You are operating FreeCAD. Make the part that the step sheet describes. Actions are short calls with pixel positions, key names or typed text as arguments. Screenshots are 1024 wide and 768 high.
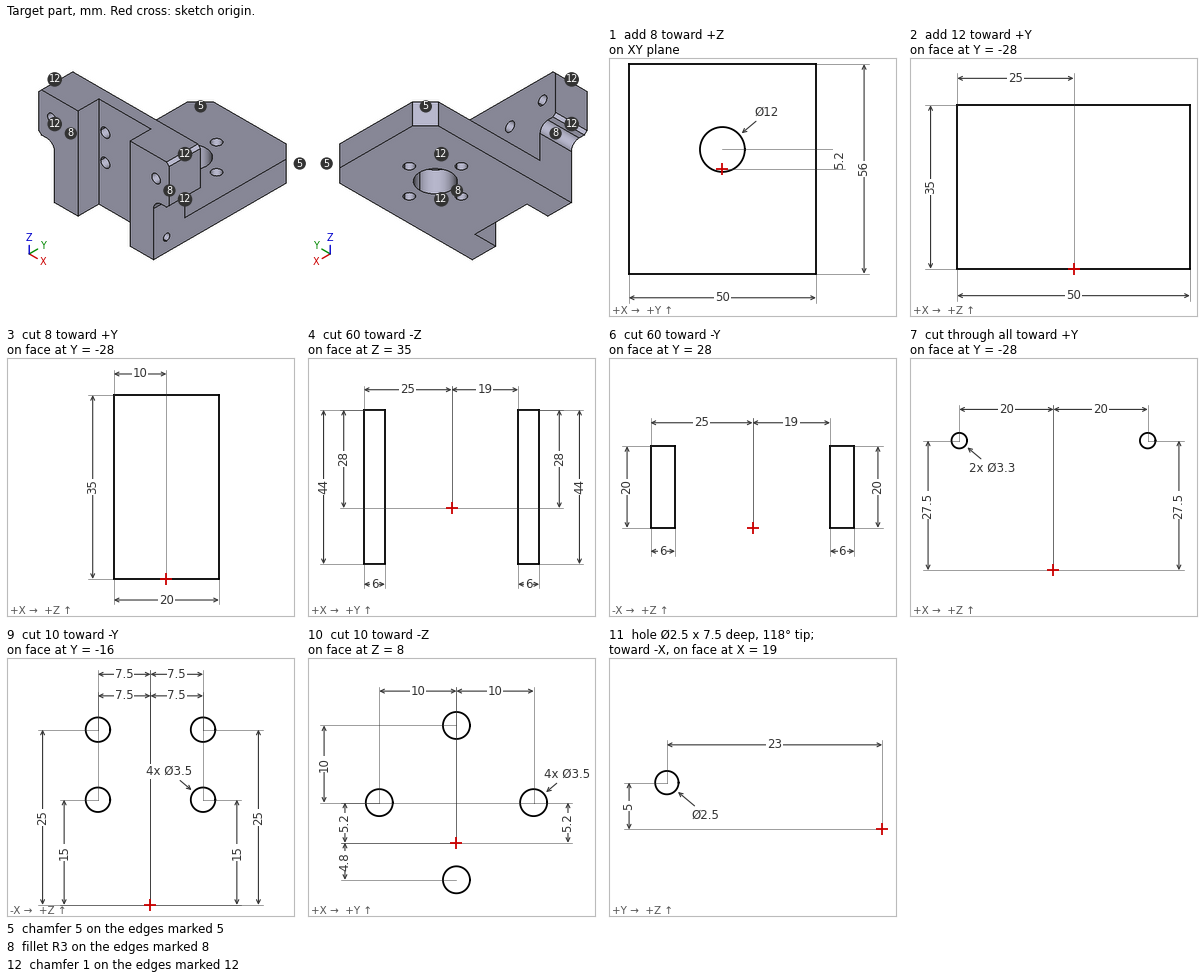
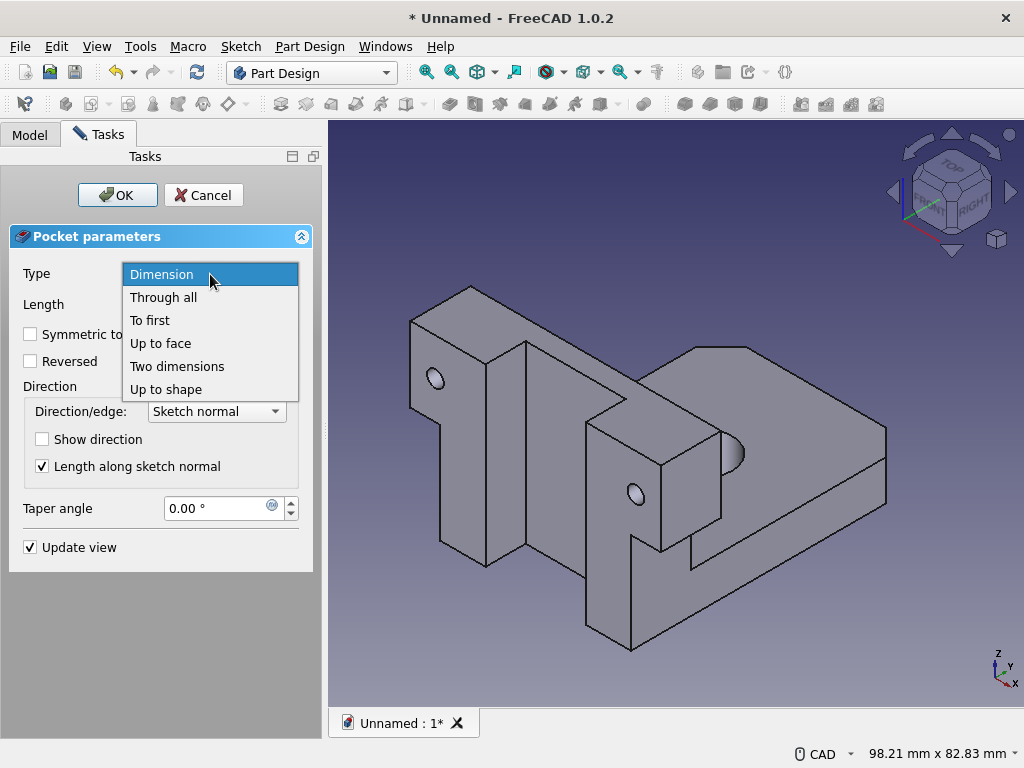
click(208, 298)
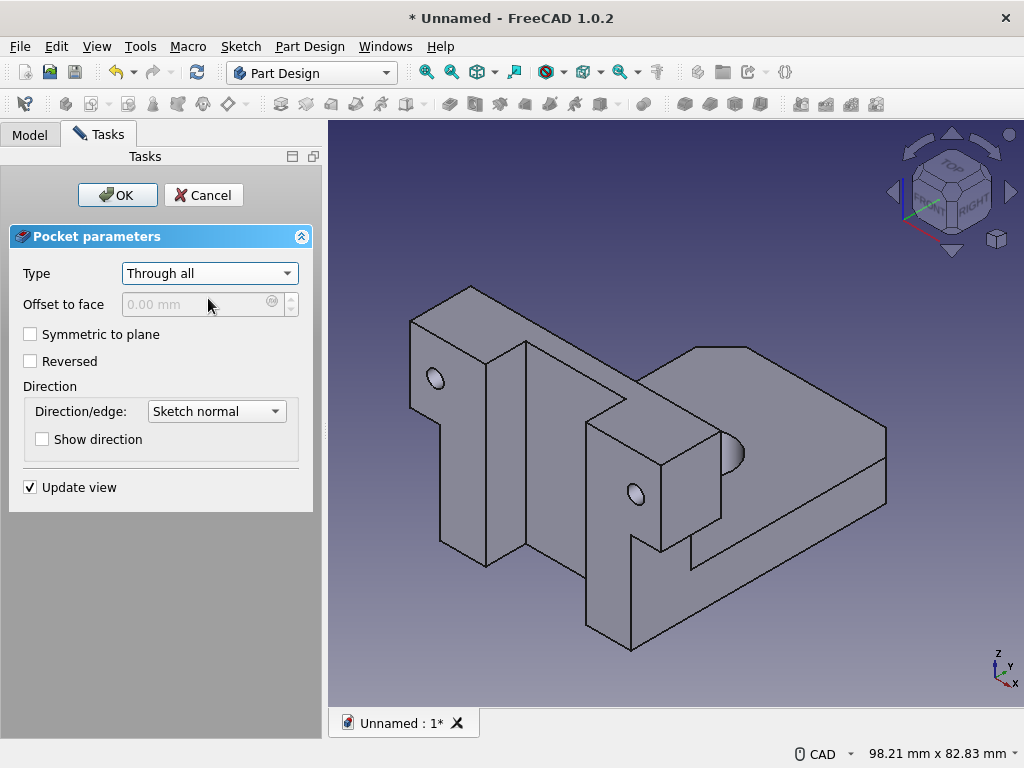
click(118, 195)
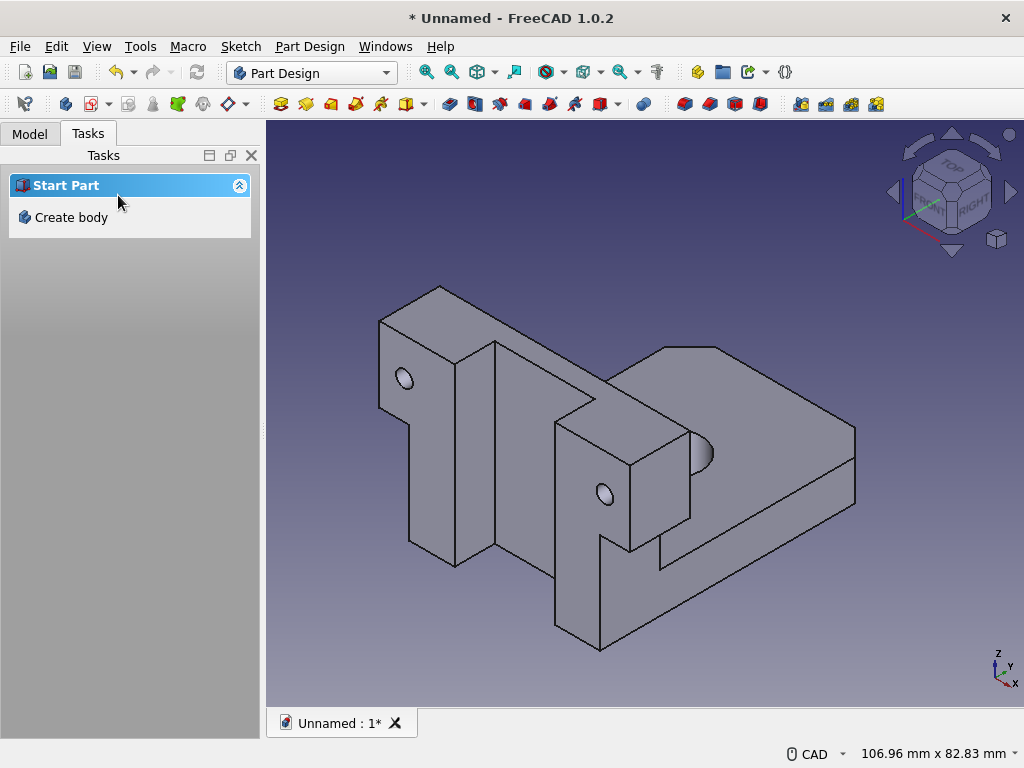
key(2)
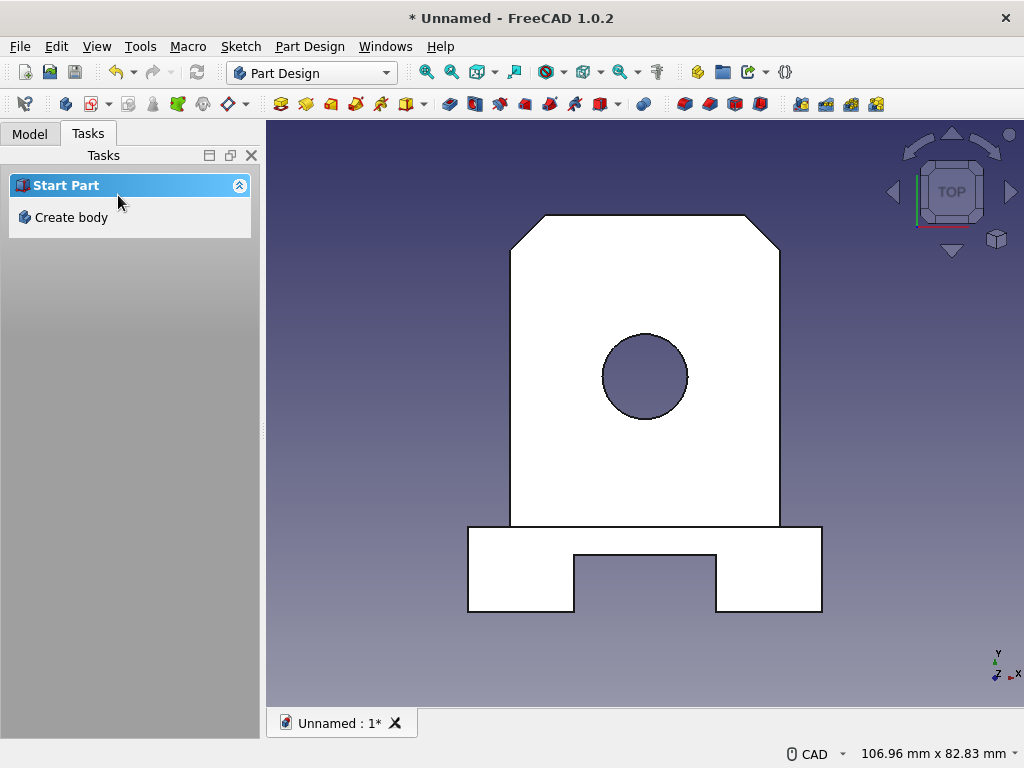
key(0)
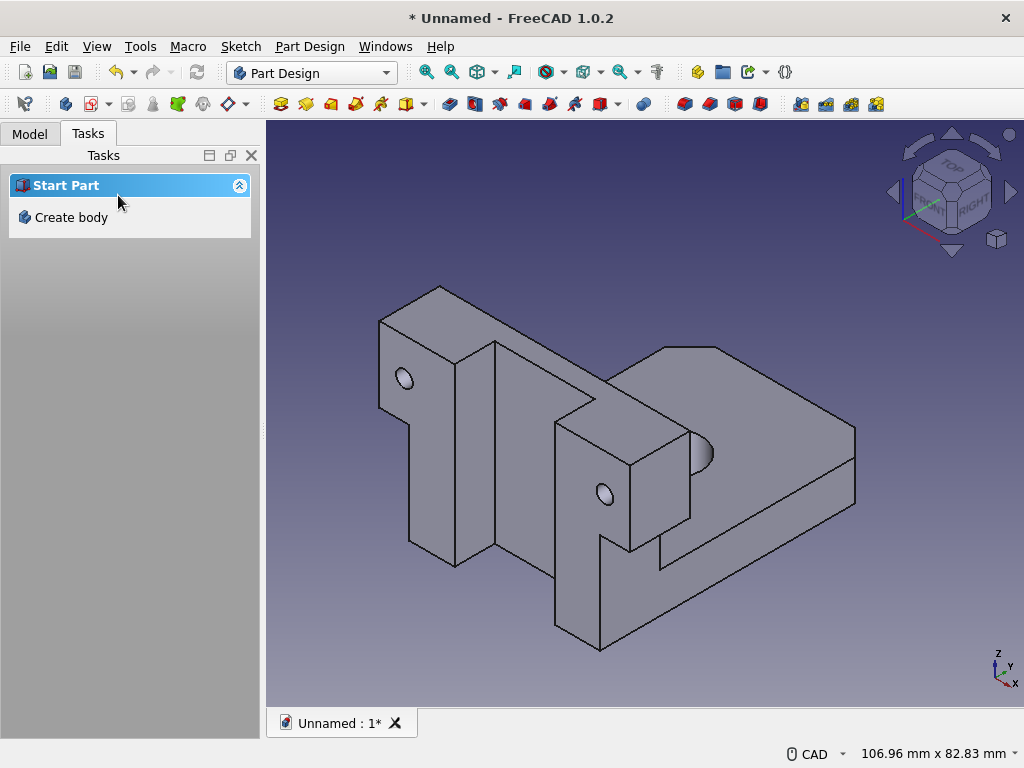
key(1)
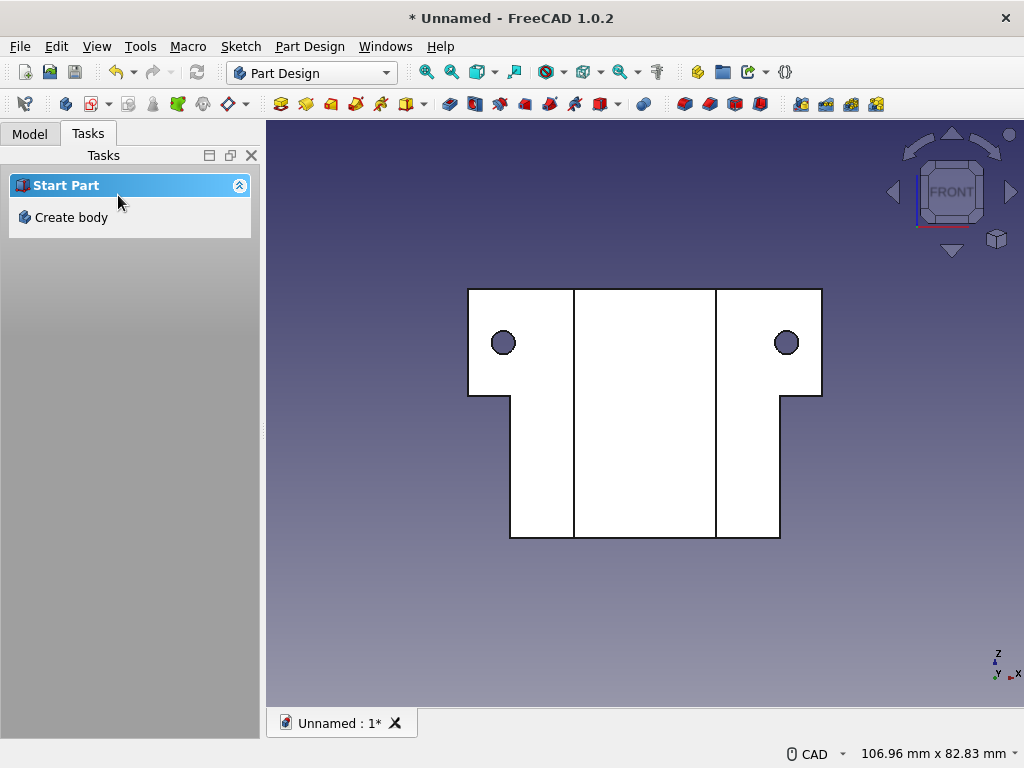
key(3)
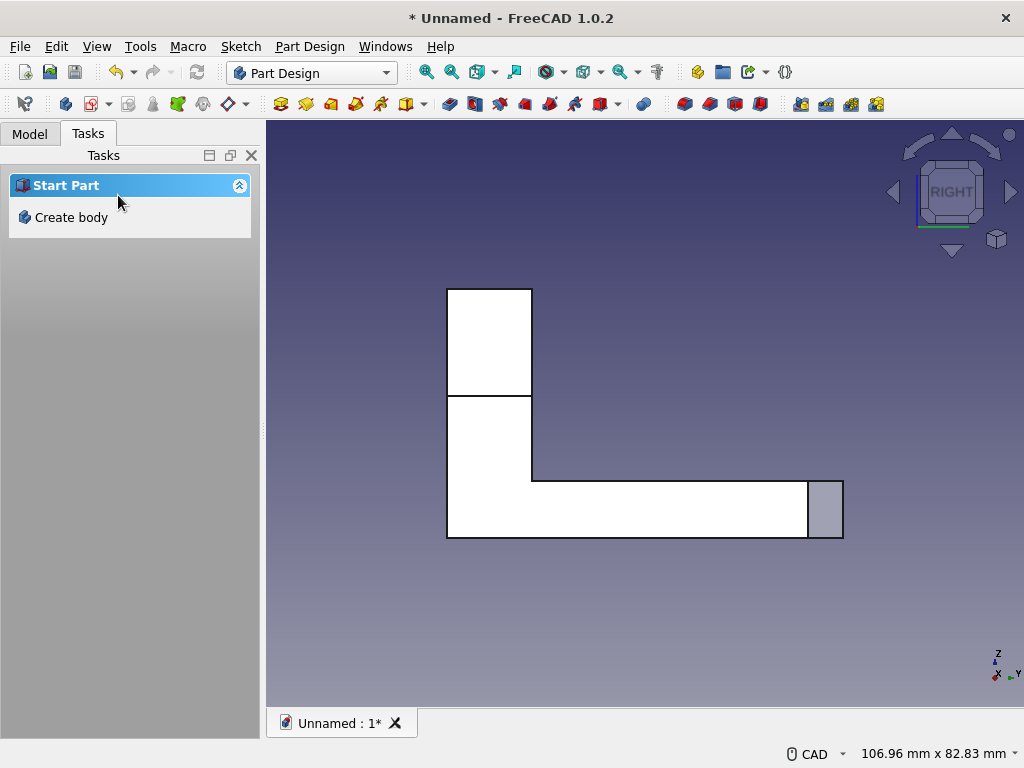
key(5)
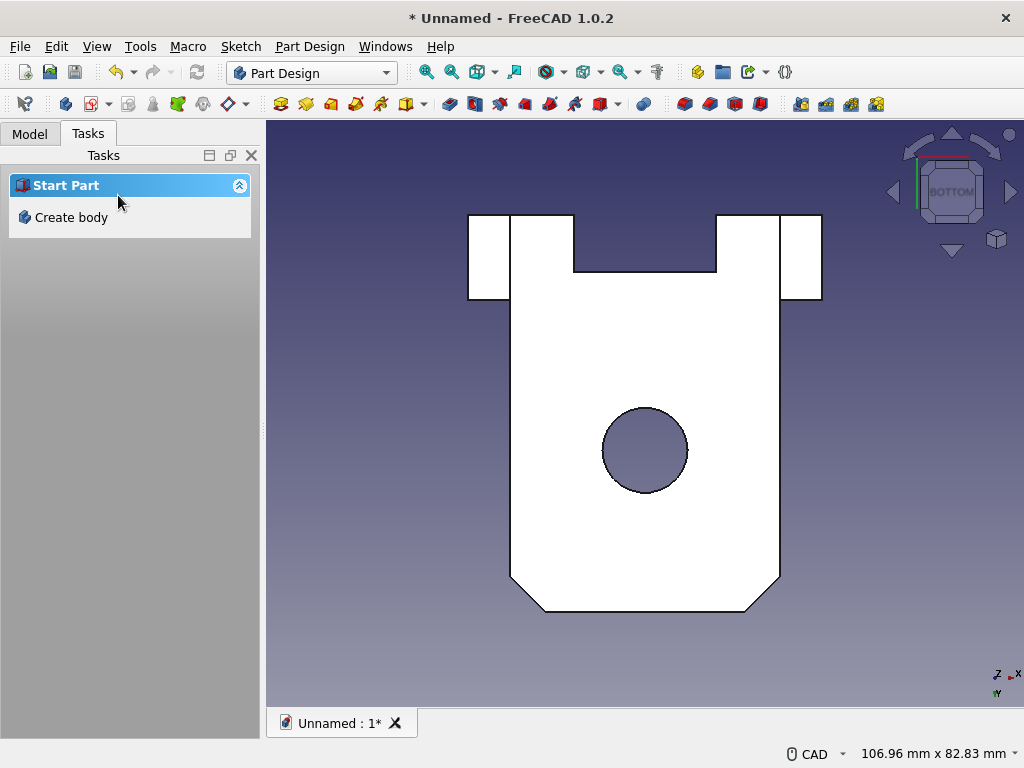
key(4)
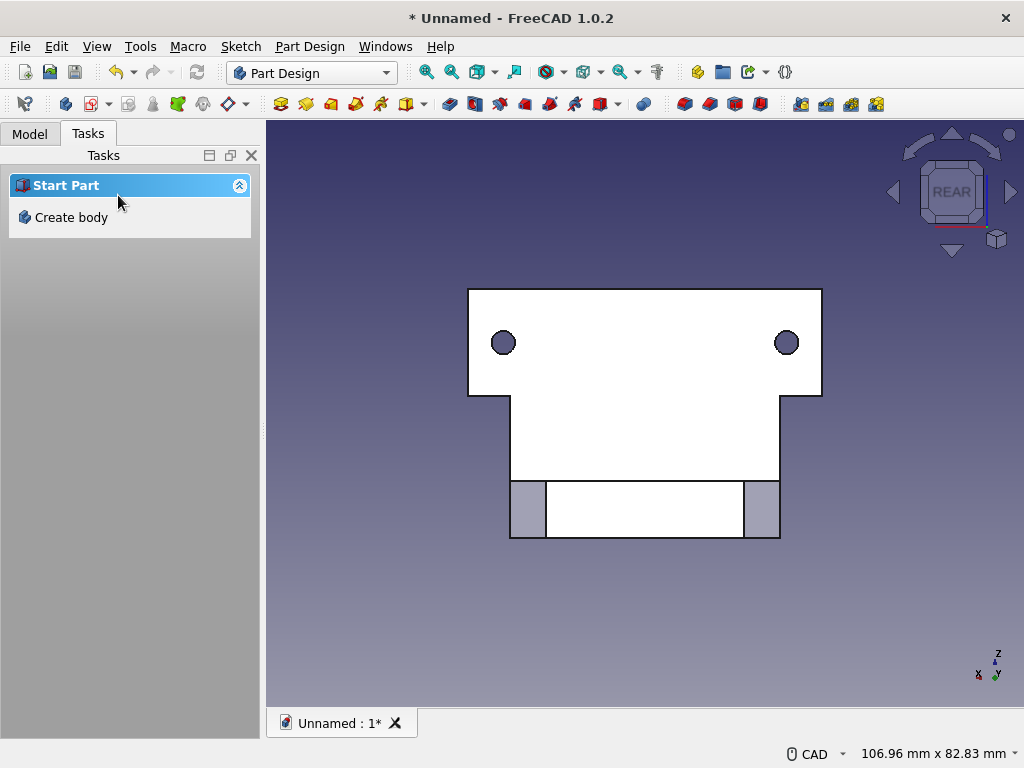
key(6)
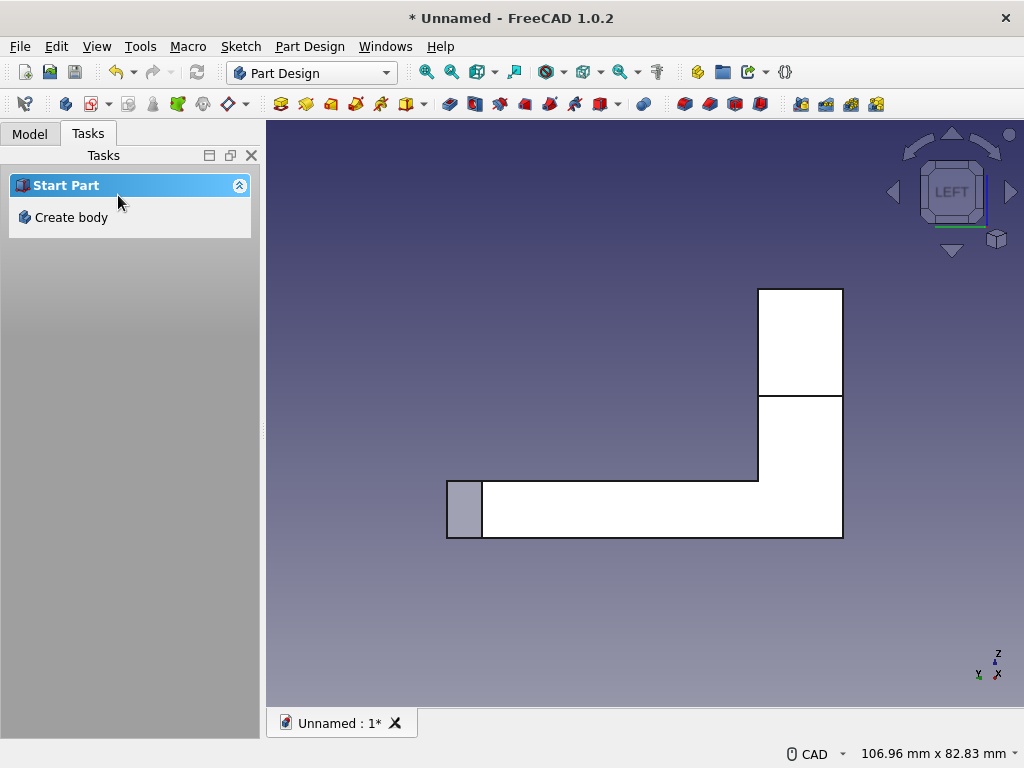
key(v)
key(3)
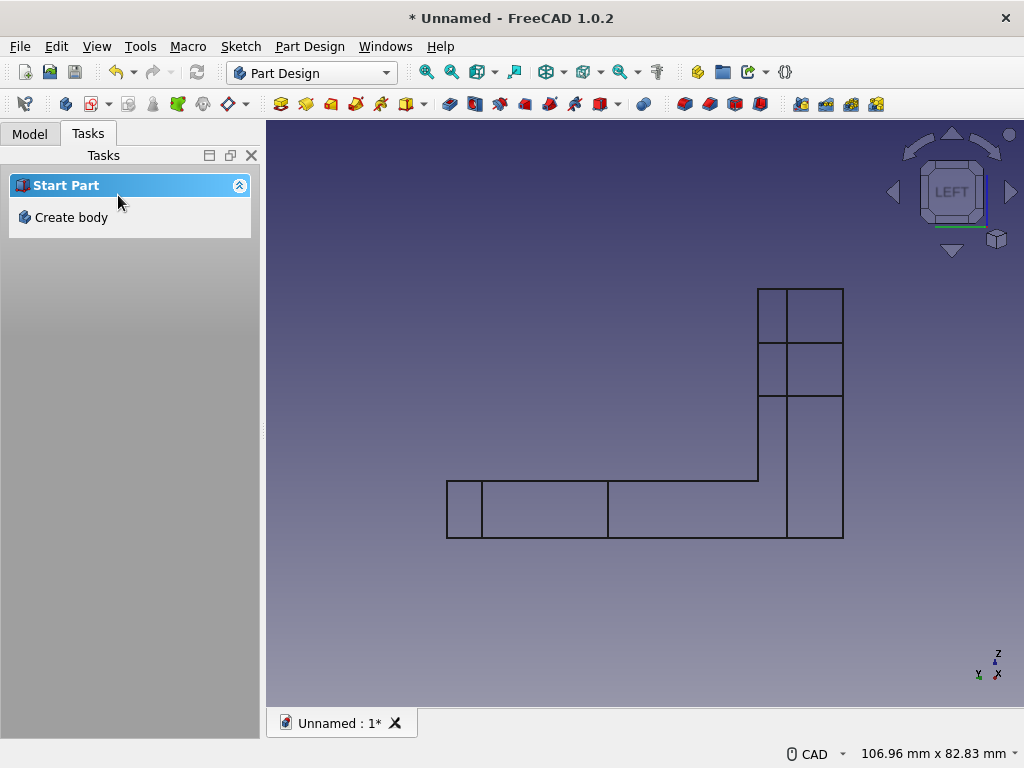
key(0)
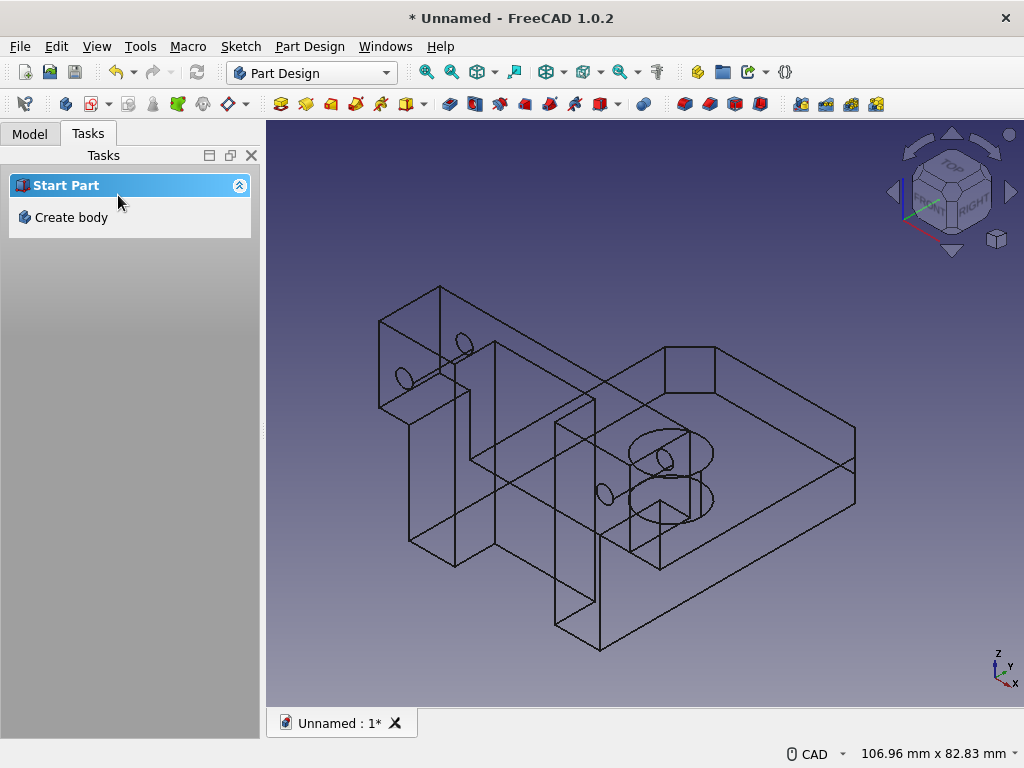
click(440, 407)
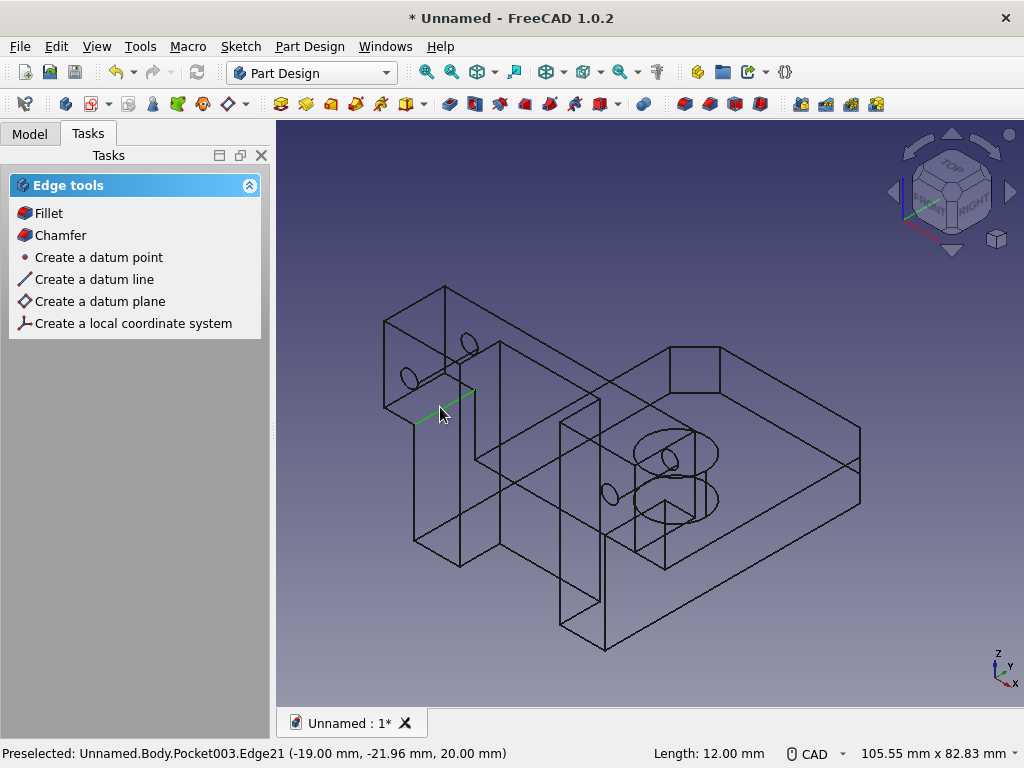
click(641, 513, ctrl)